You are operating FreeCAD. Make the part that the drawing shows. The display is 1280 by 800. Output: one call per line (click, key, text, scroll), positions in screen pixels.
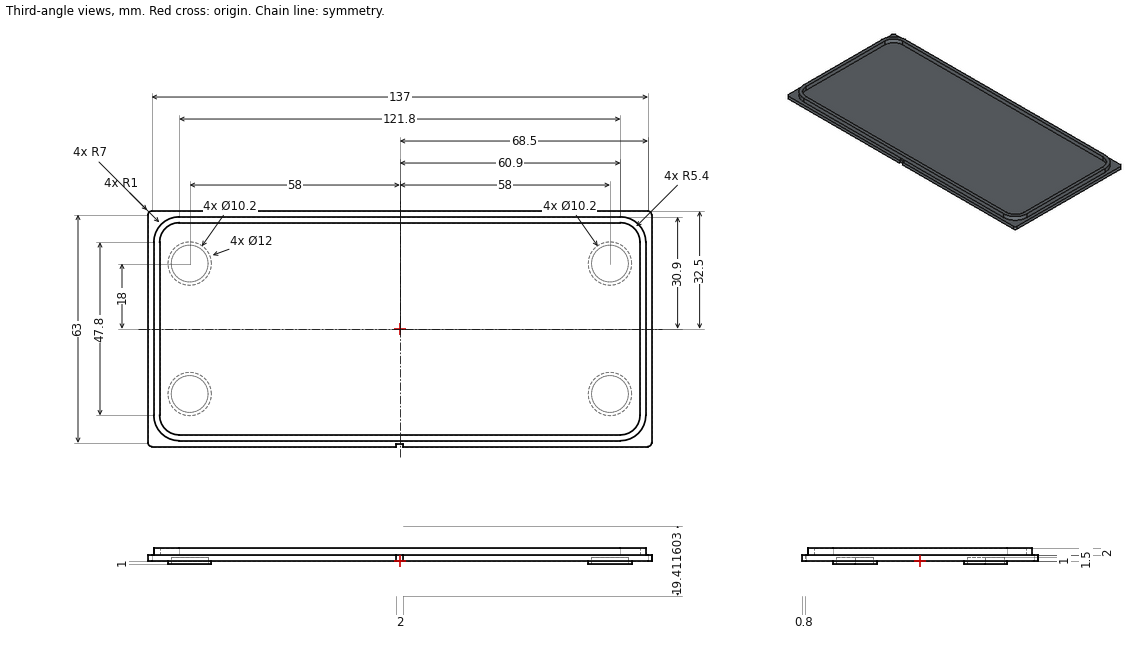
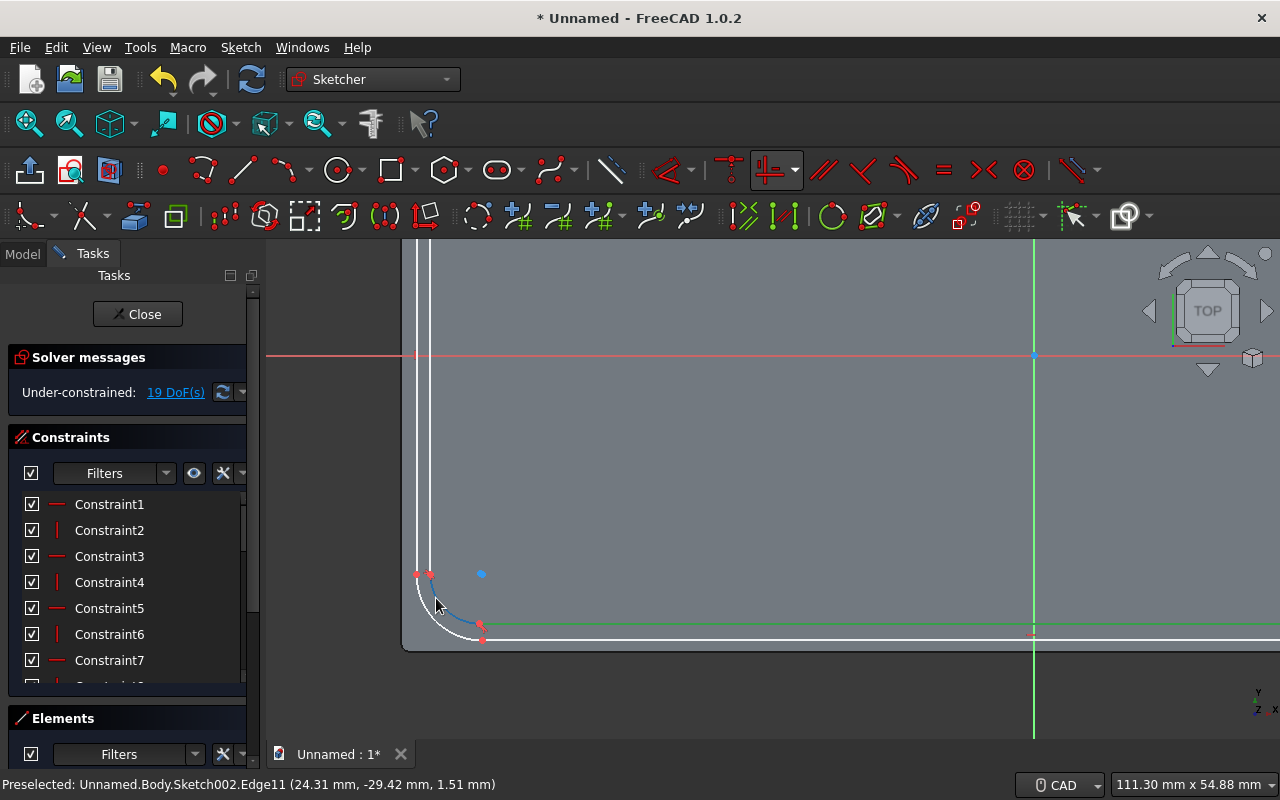
click(436, 597)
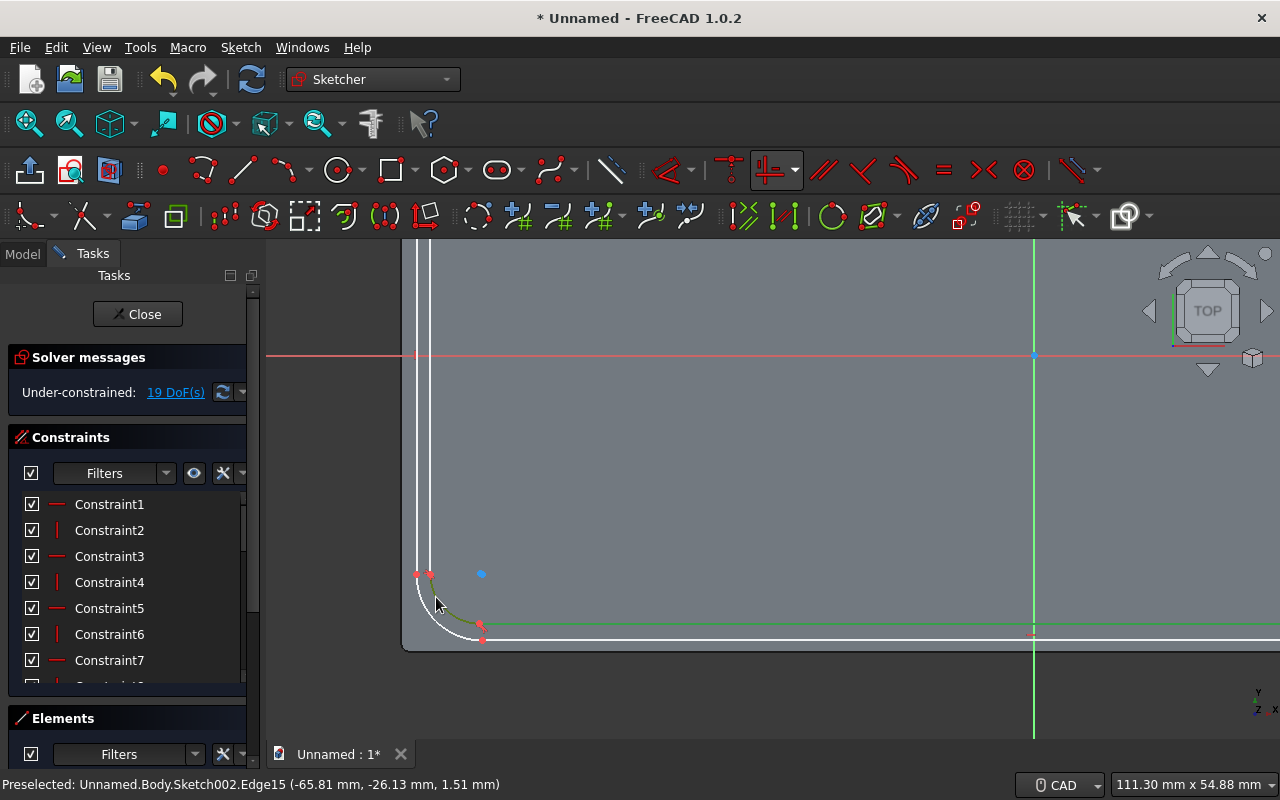
click(904, 170)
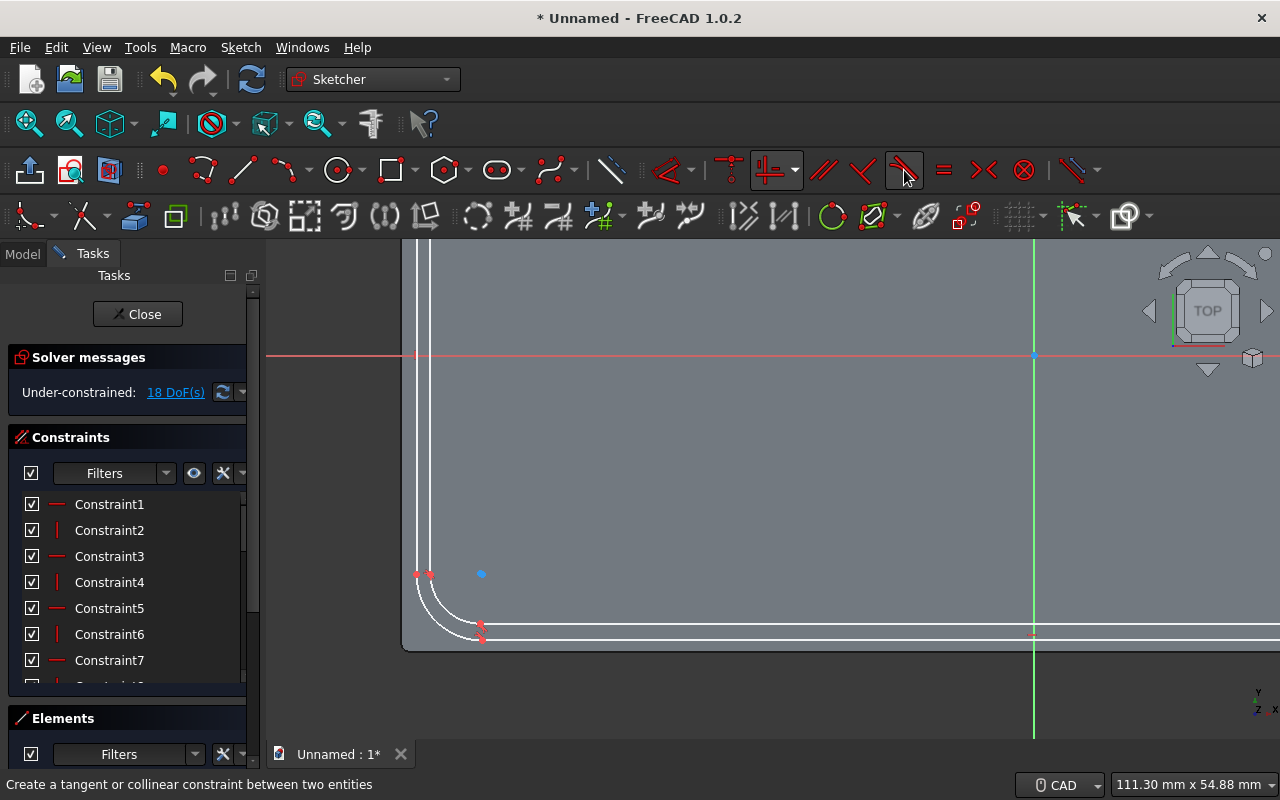
click(430, 444)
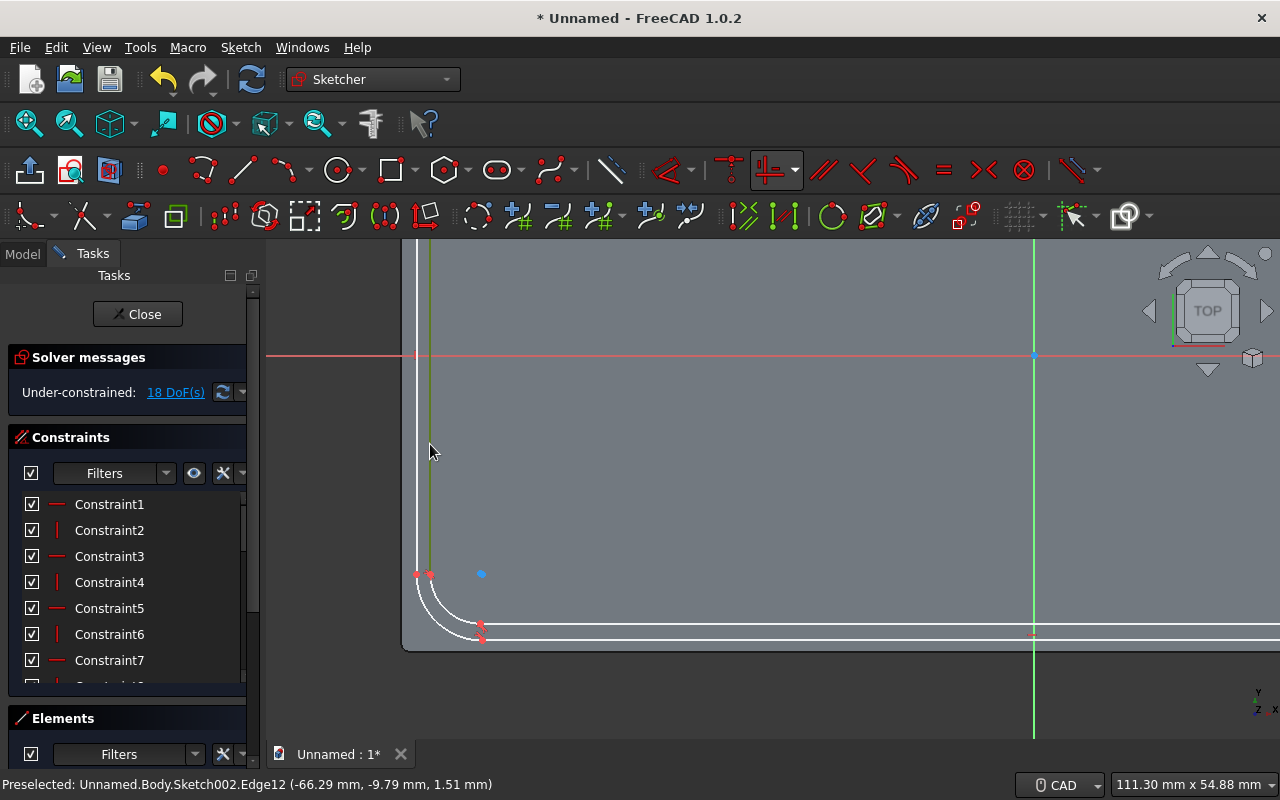
click(436, 597)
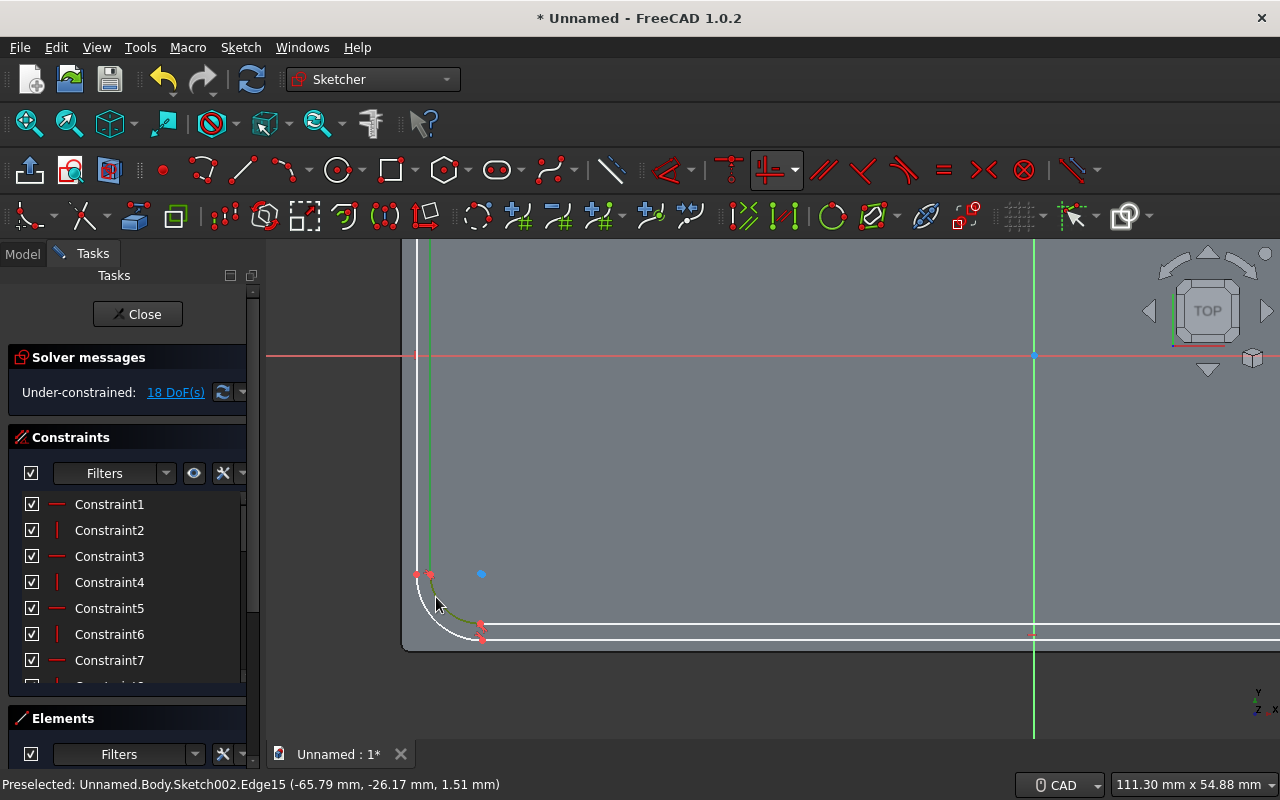
click(904, 170)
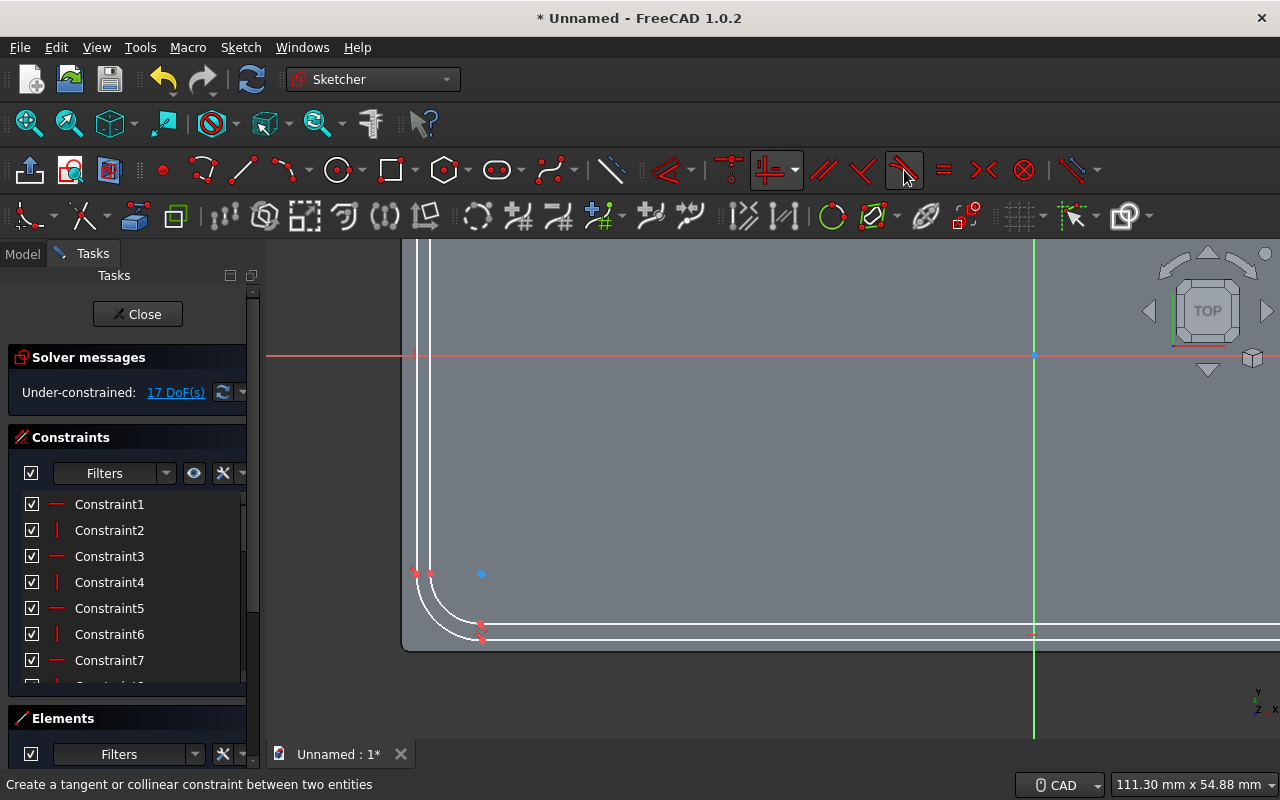
click(430, 443)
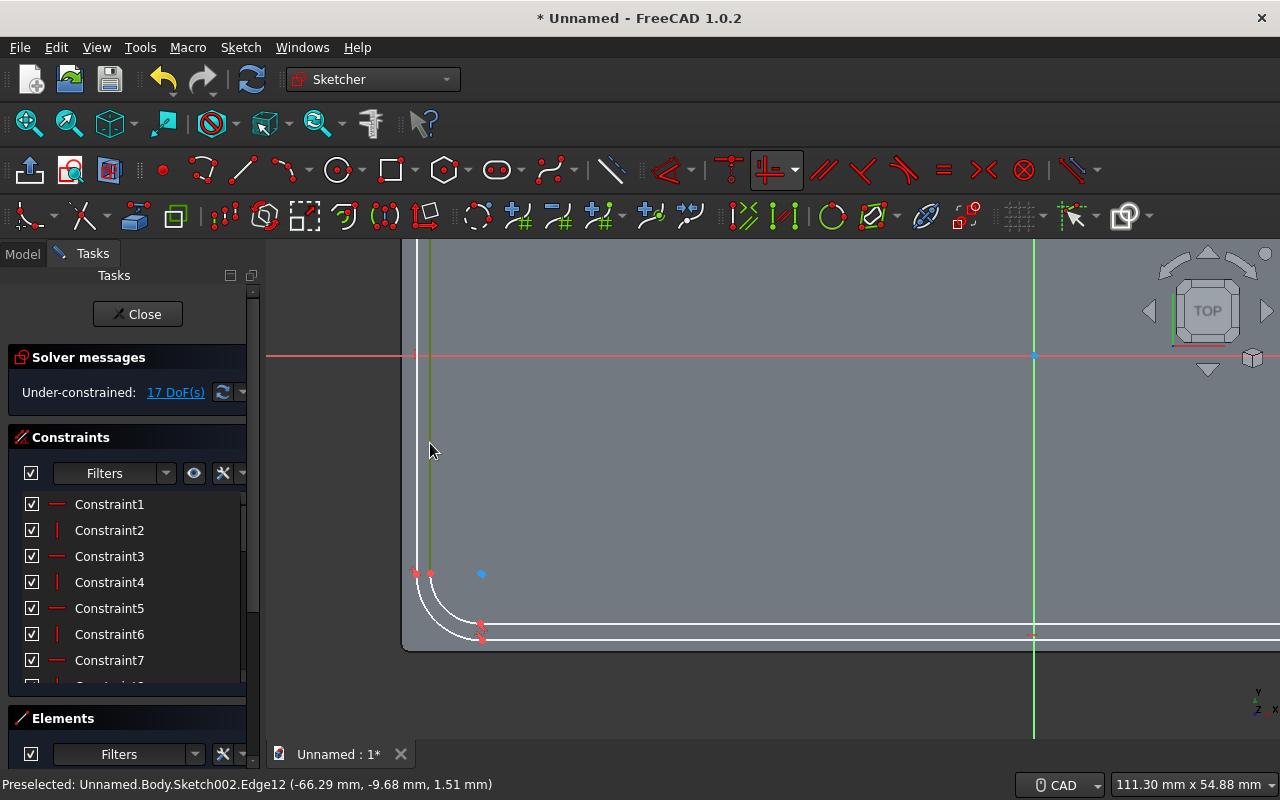
scroll(435, 598, down, 4)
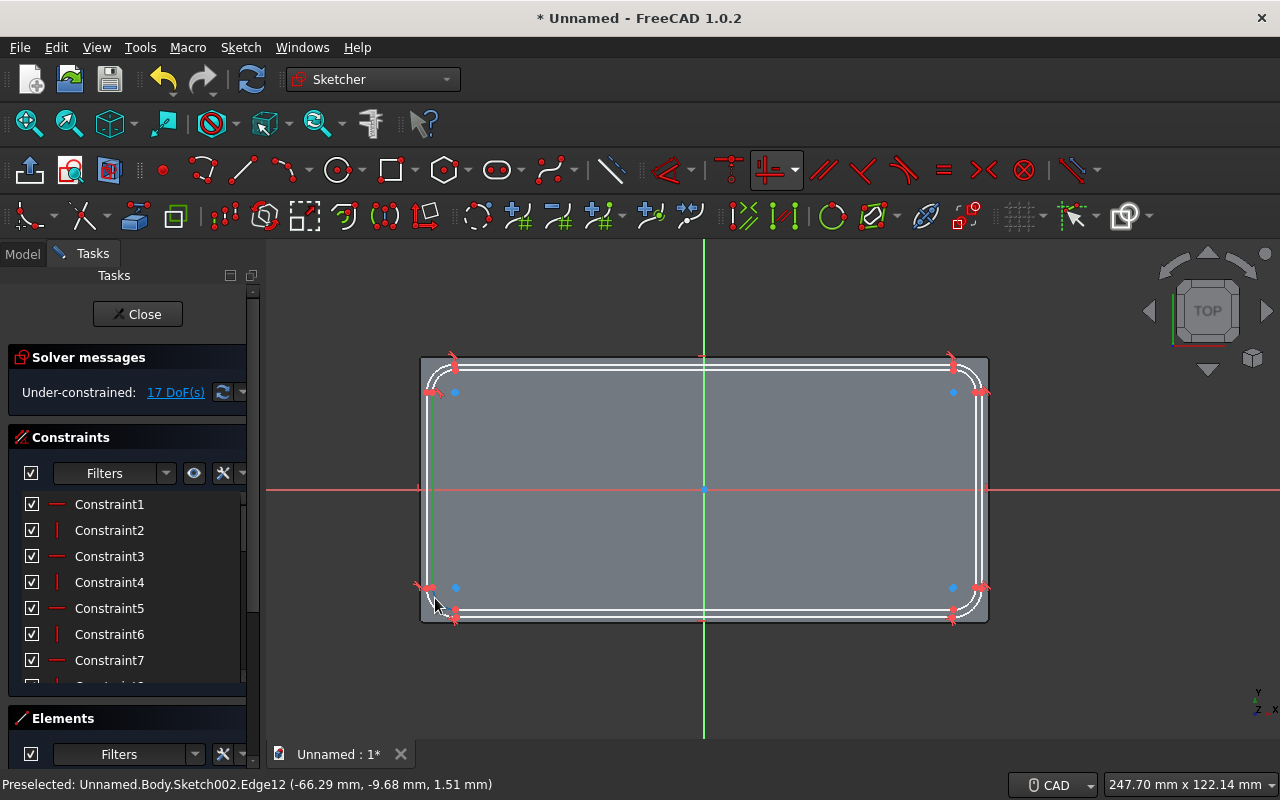
scroll(445, 372, up, 5)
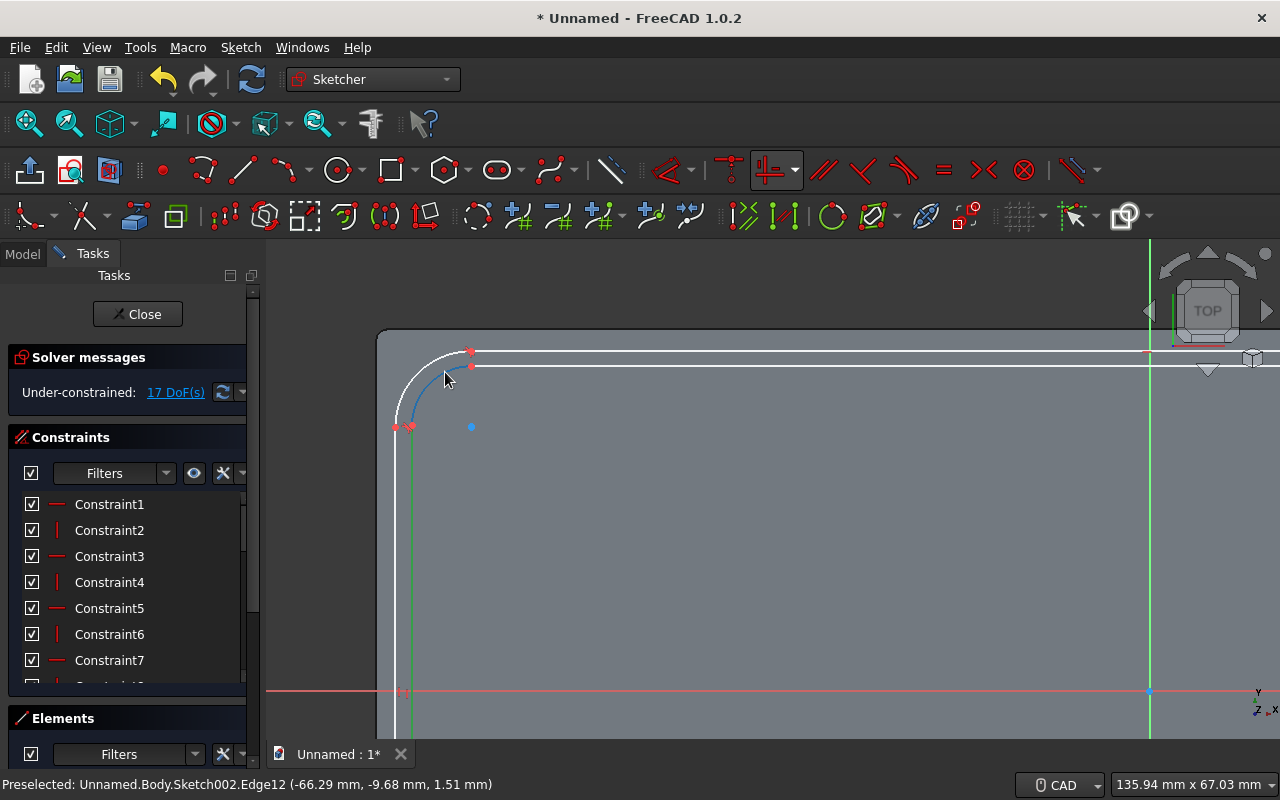
click(445, 373)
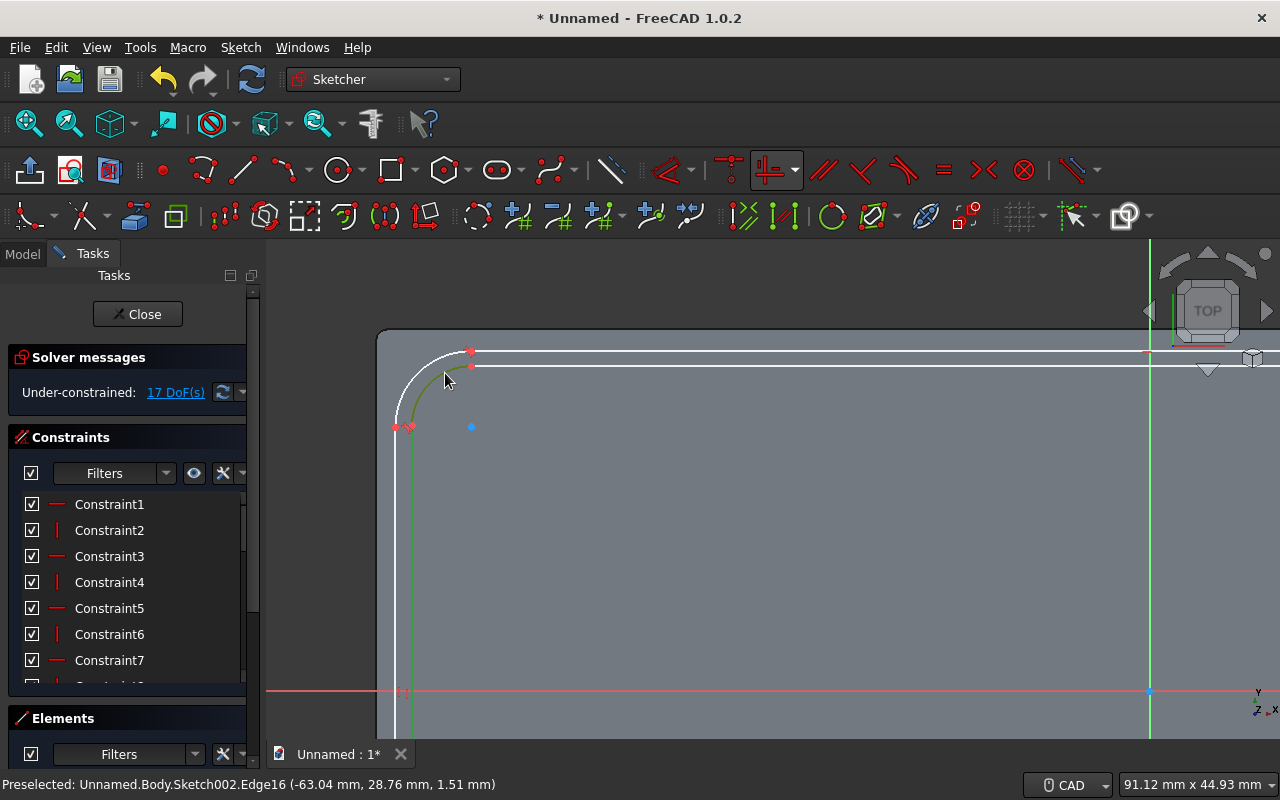
click(904, 170)